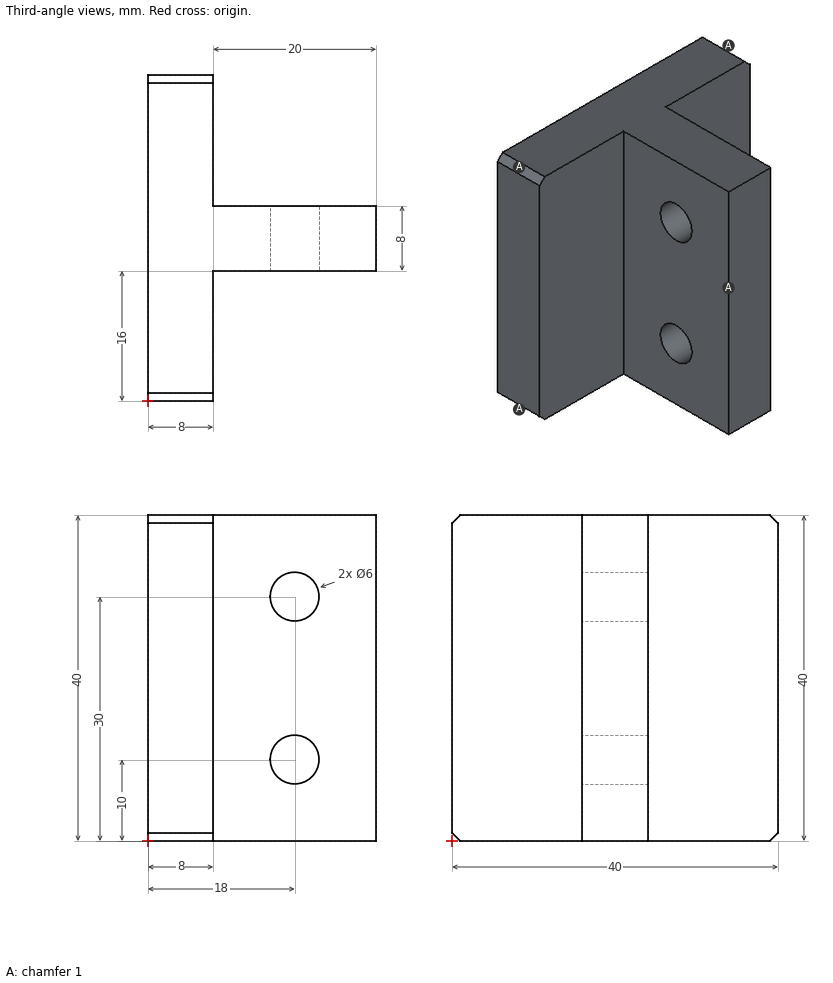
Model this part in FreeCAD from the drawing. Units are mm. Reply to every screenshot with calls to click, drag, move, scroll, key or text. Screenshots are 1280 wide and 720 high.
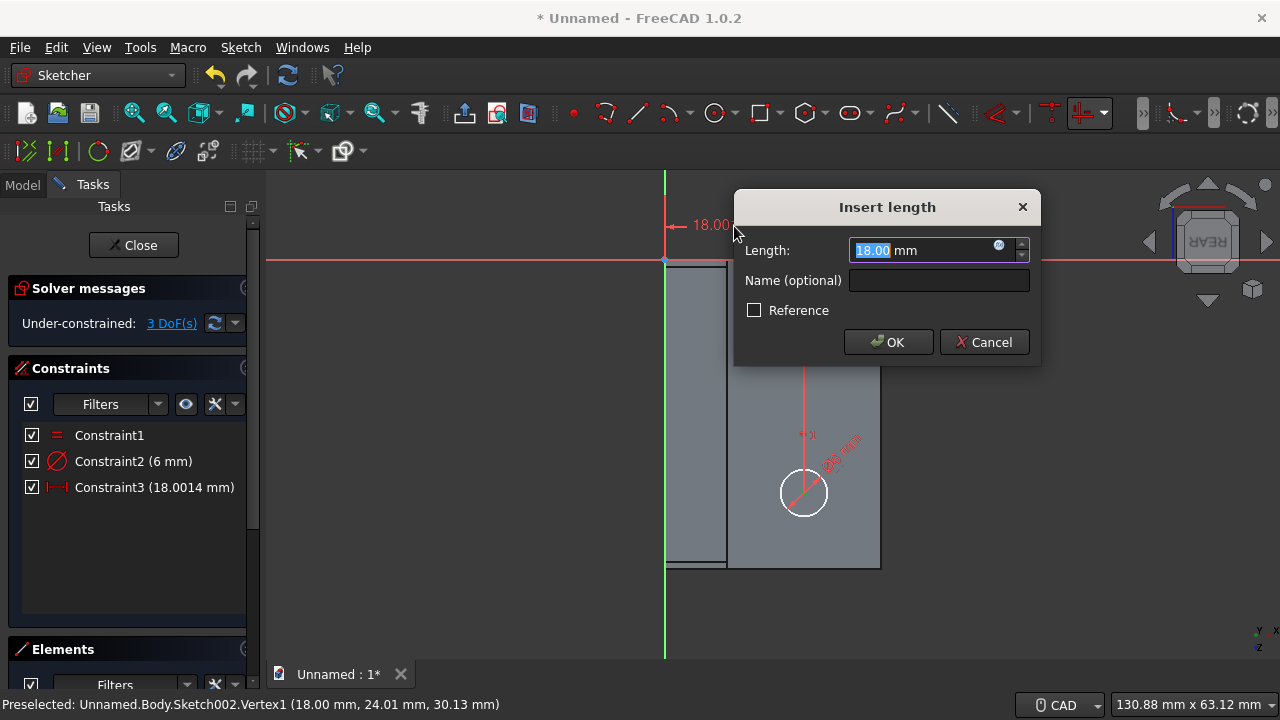
text(18)
key(Return)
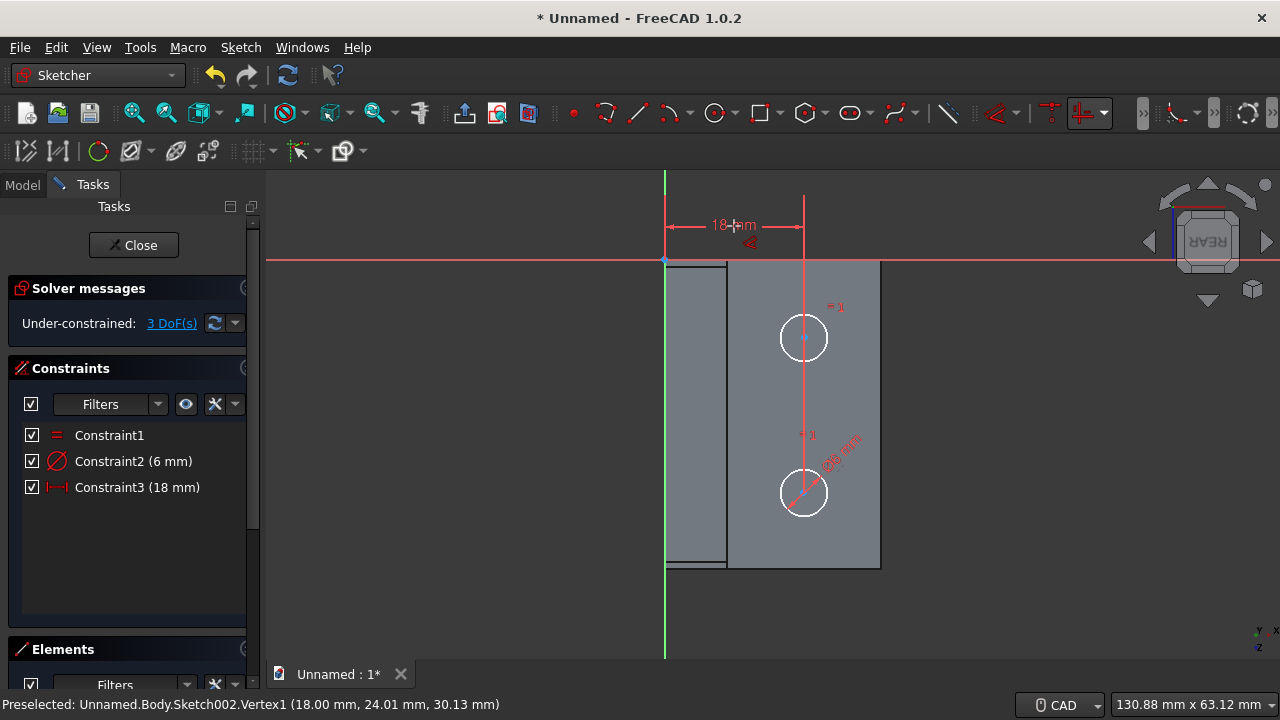
click(804, 493)
click(631, 376)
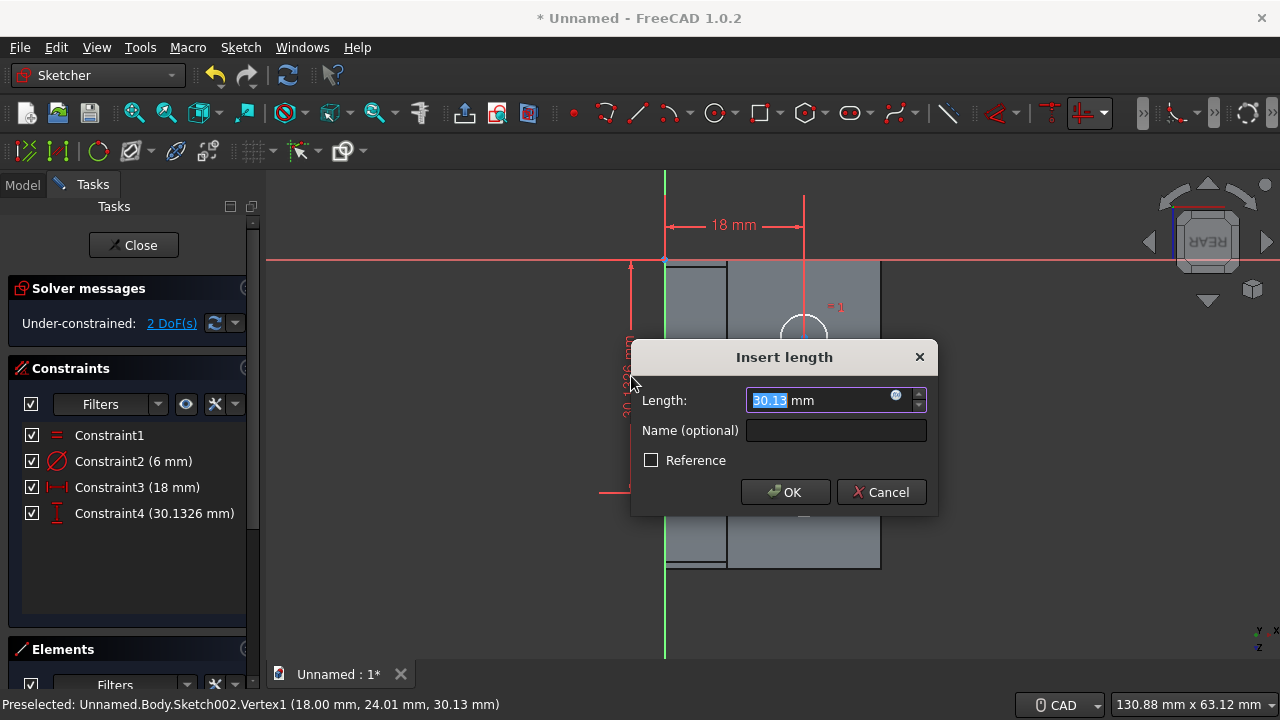
text(30)
key(Return)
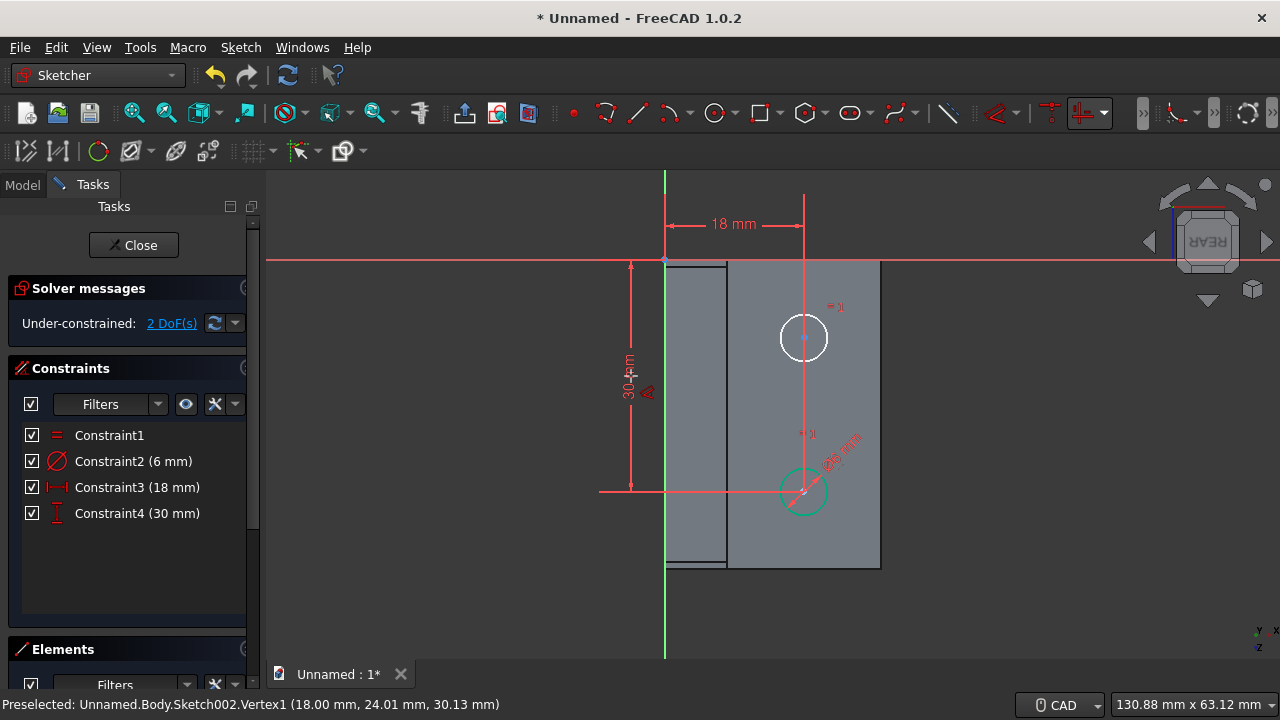
click(804, 338)
click(734, 372)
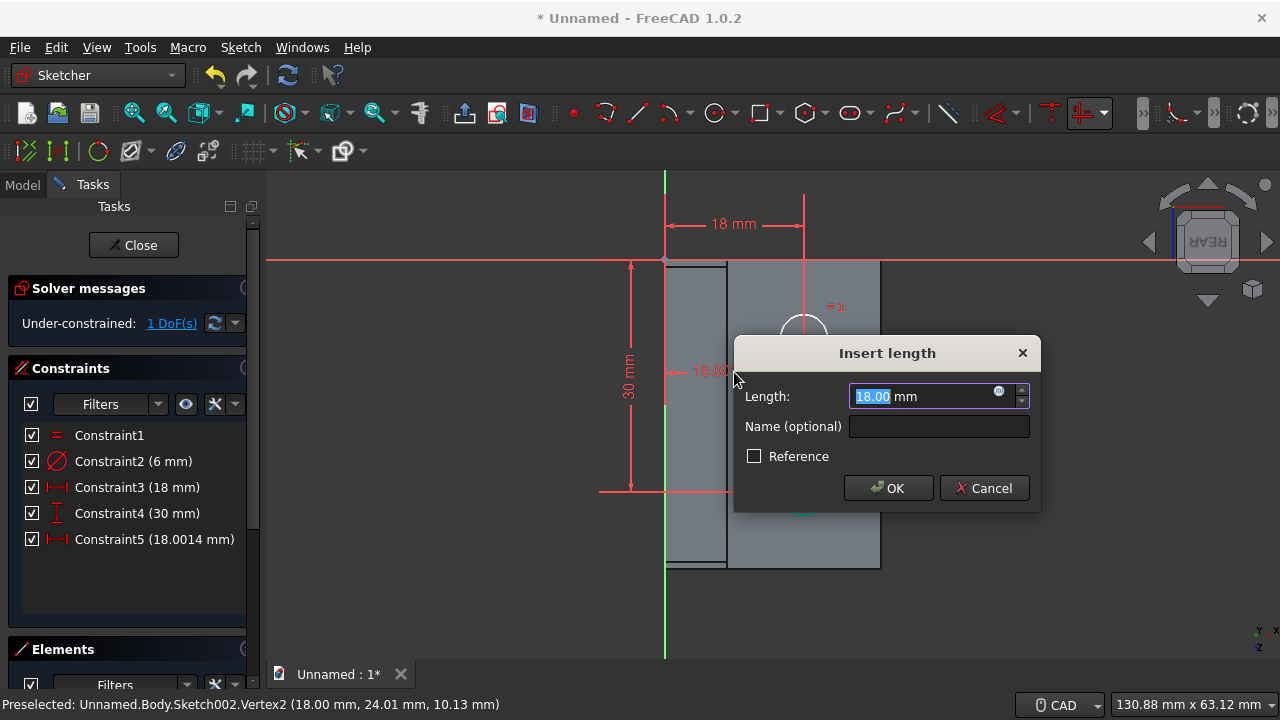
text(18)
key(Return)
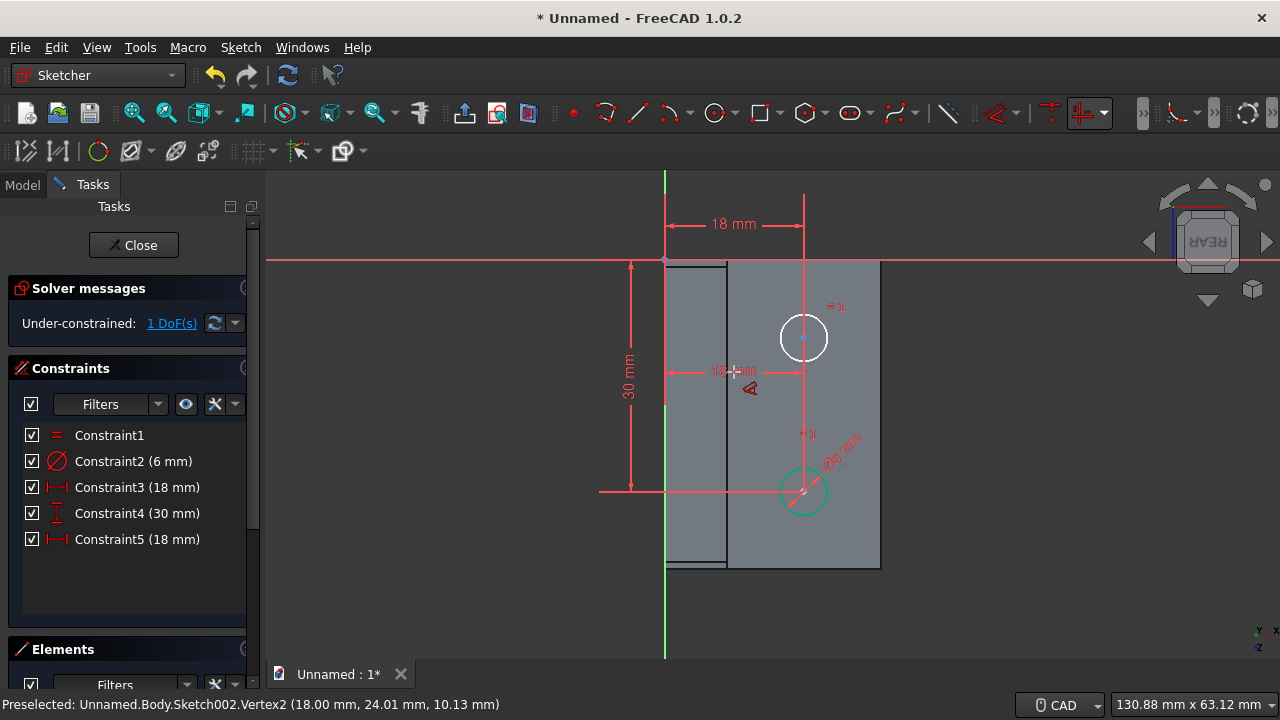
click(804, 338)
click(631, 299)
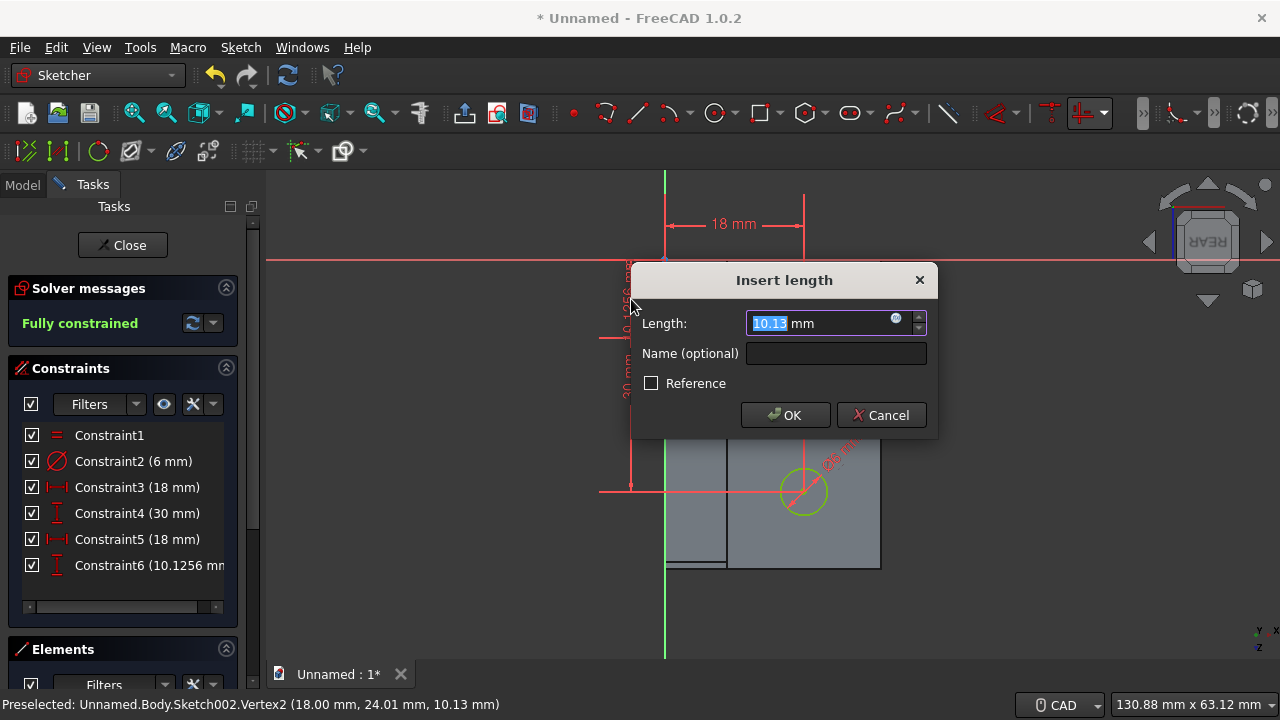
text(10)
key(Return)
key(Escape)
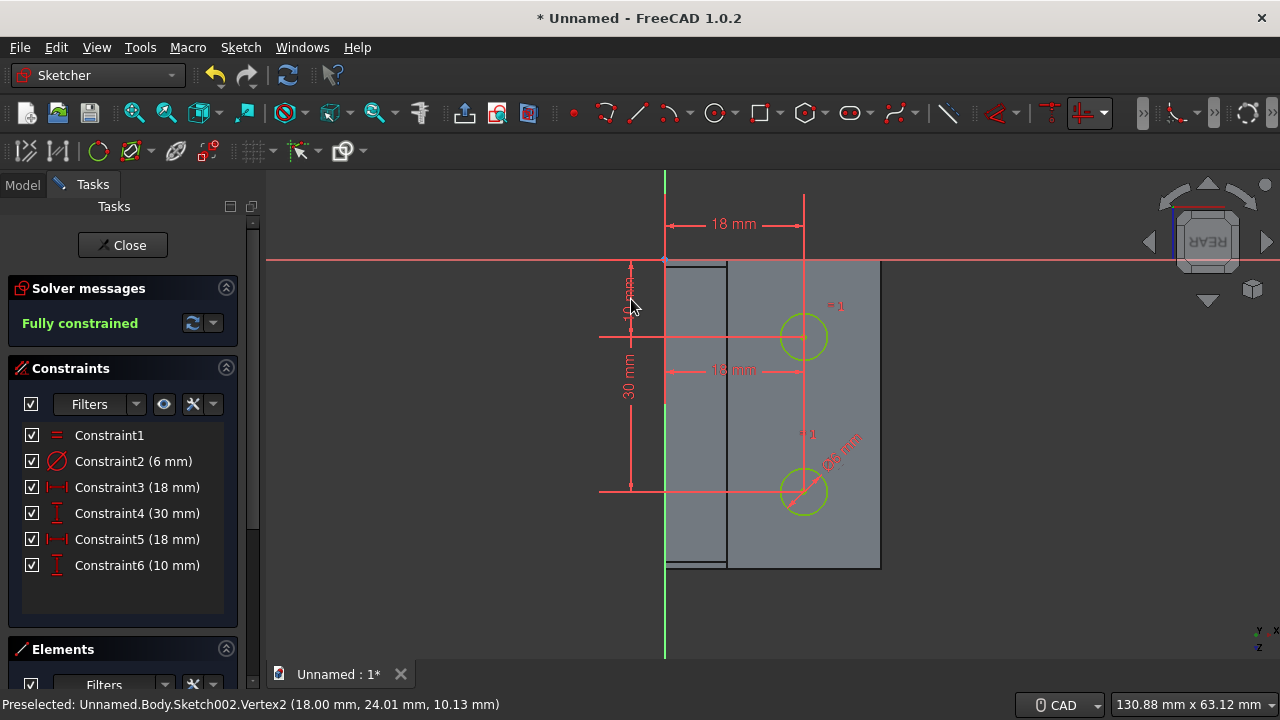
click(123, 245)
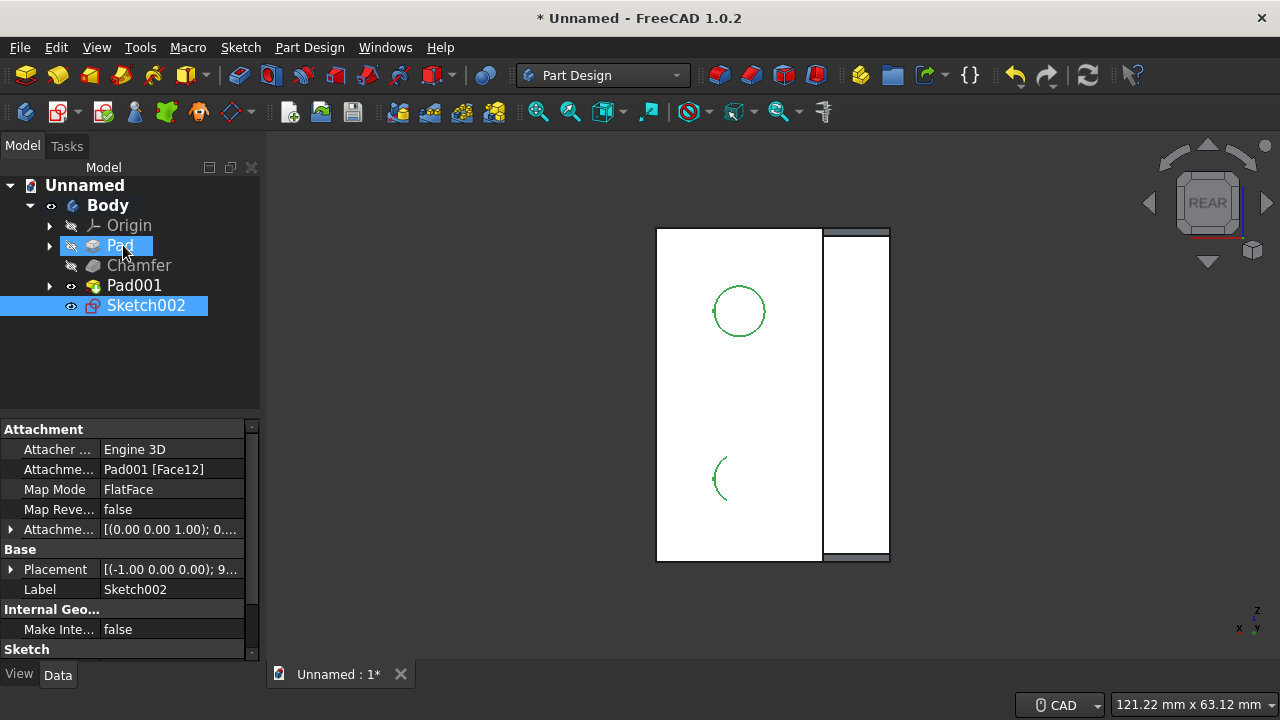
click(240, 76)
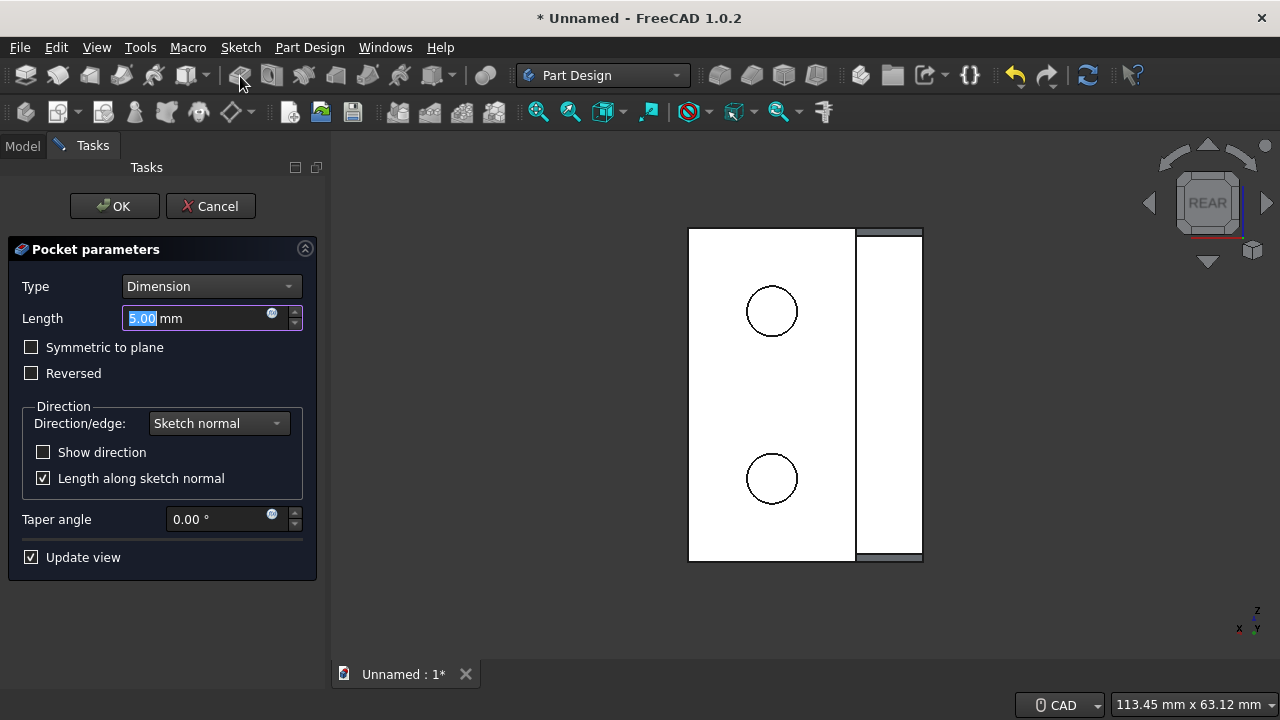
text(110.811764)
key(Tab)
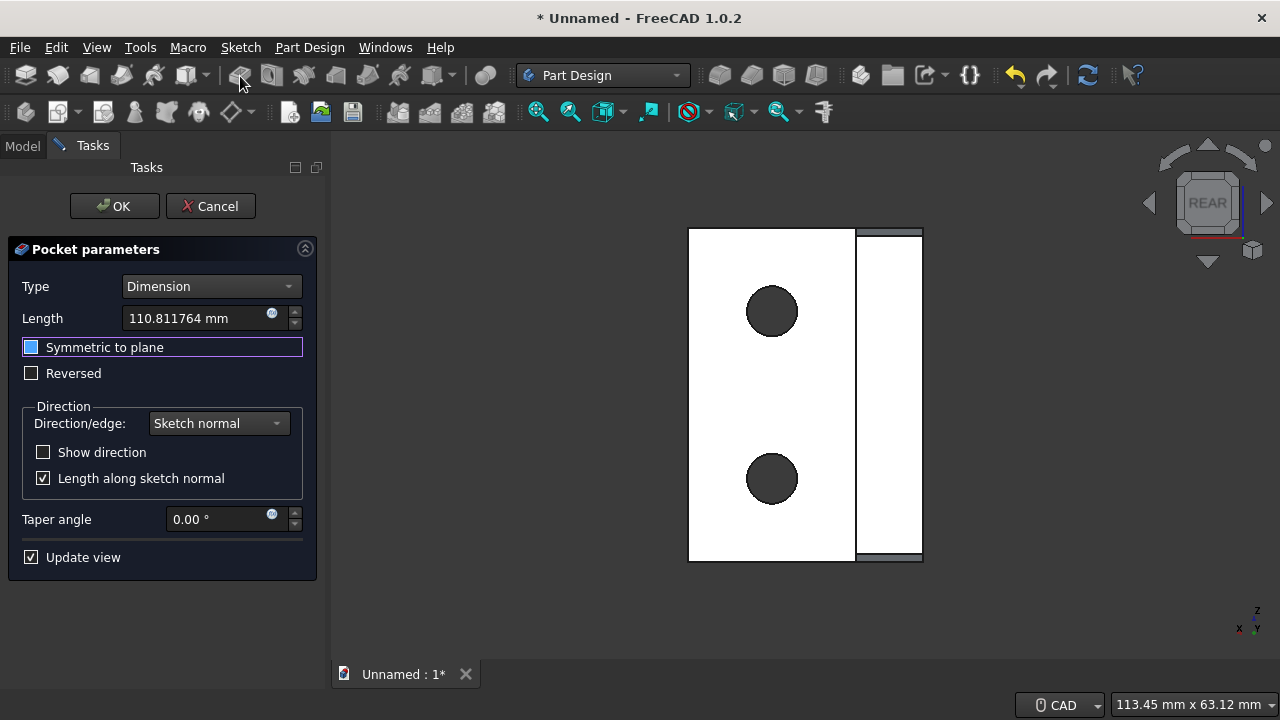
click(30, 347)